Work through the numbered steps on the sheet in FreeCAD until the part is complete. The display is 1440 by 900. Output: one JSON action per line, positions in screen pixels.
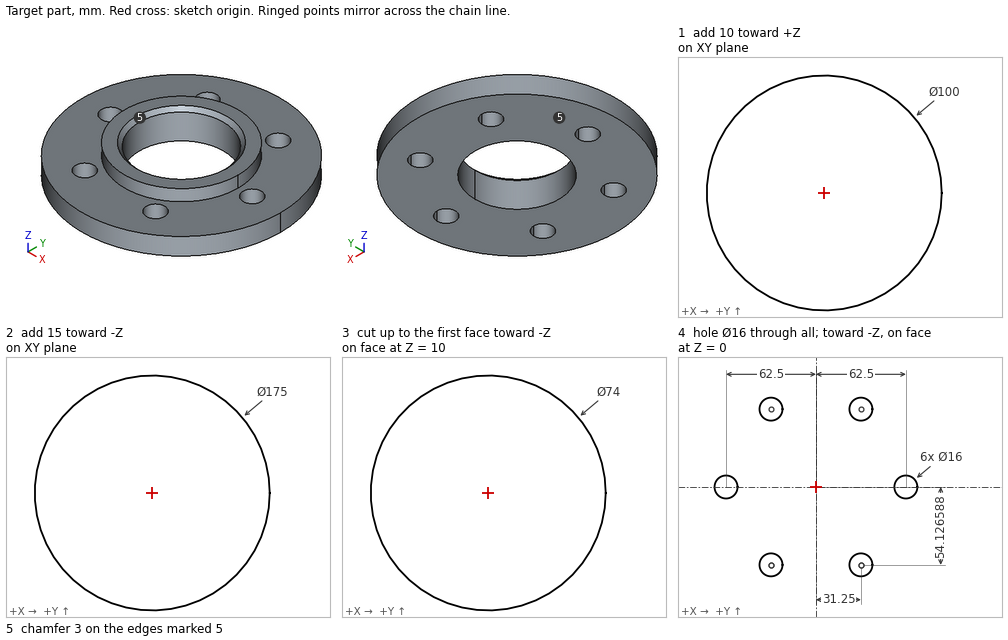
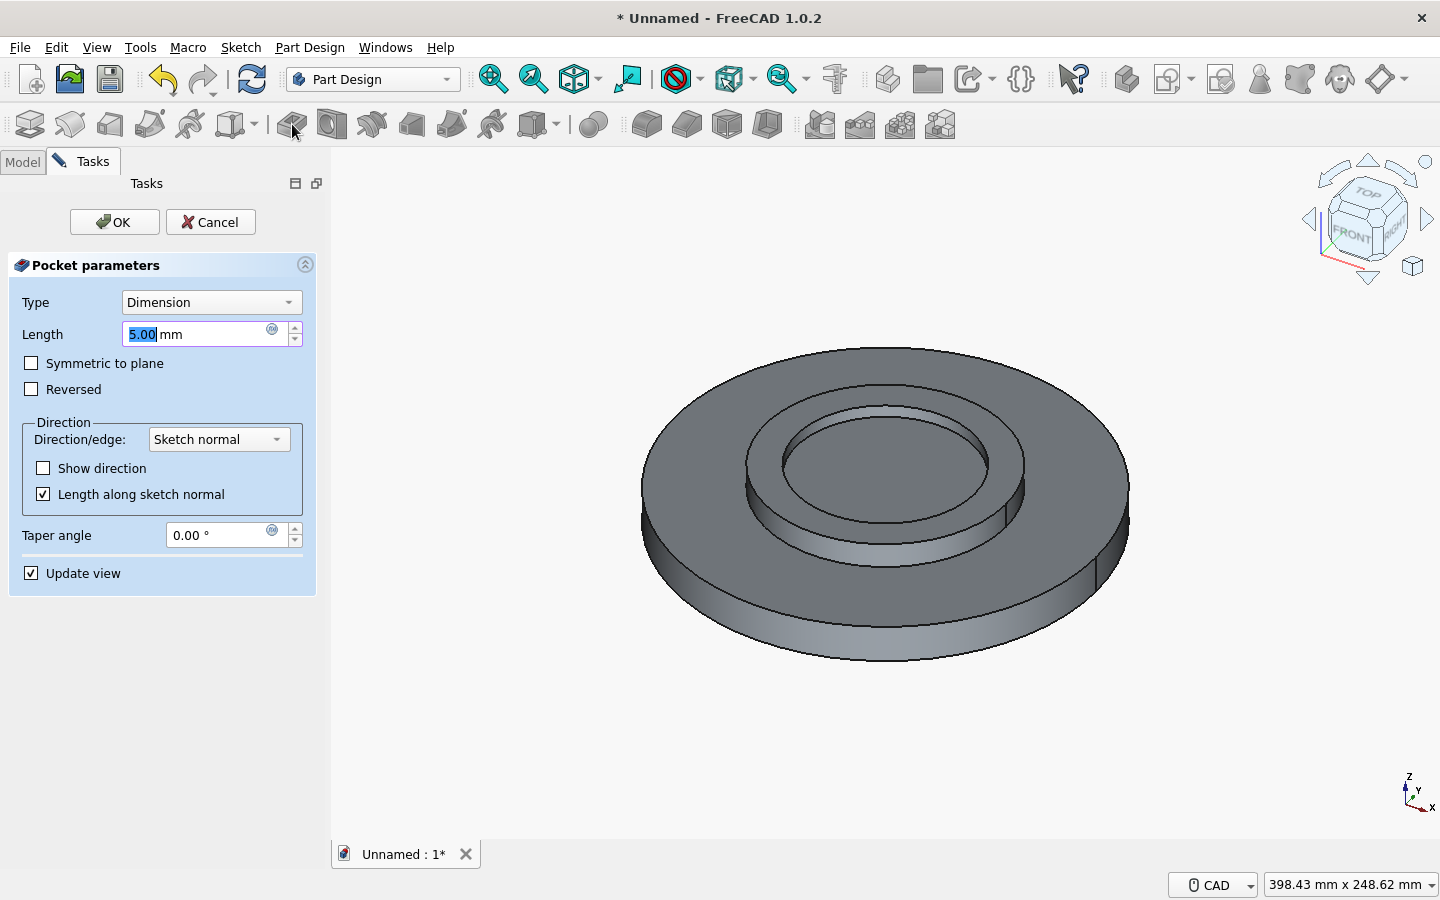
{"action": "left_click", "coordinate": [212, 302]}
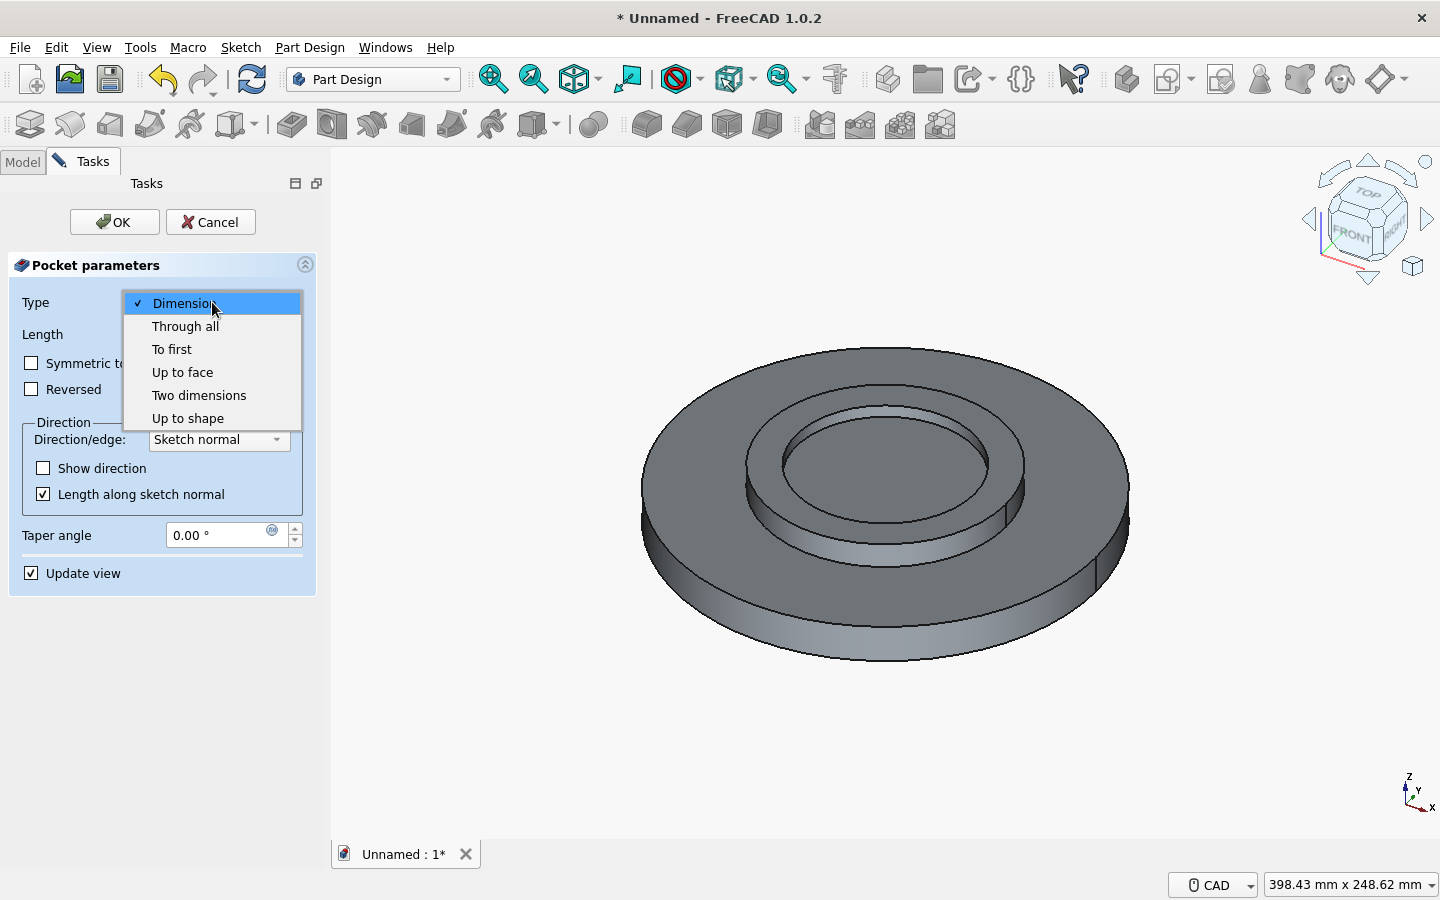
{"action": "left_click", "coordinate": [212, 350]}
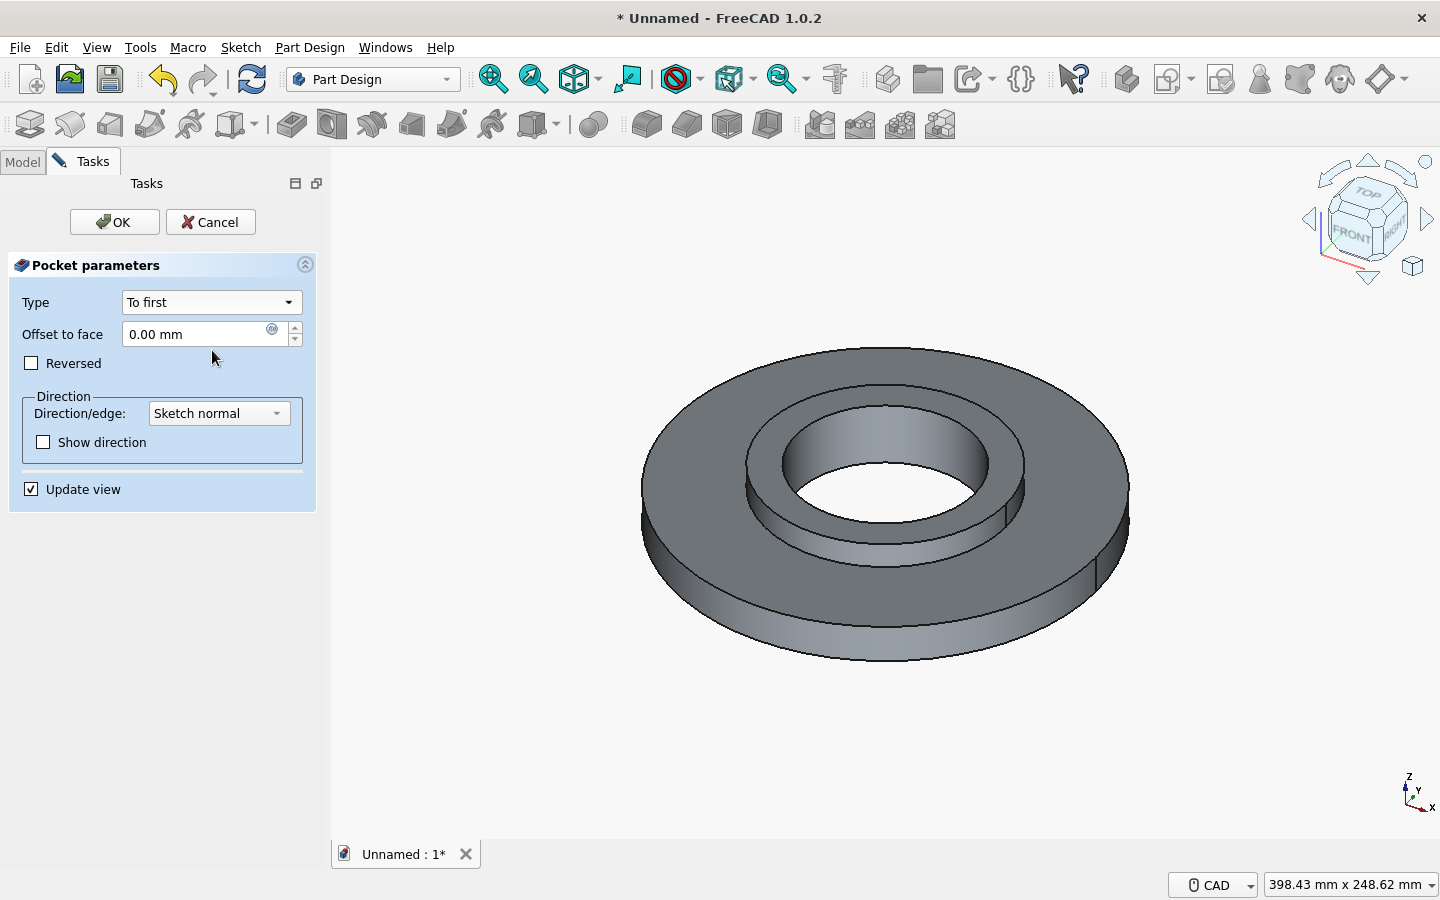
{"action": "left_click", "coordinate": [115, 222]}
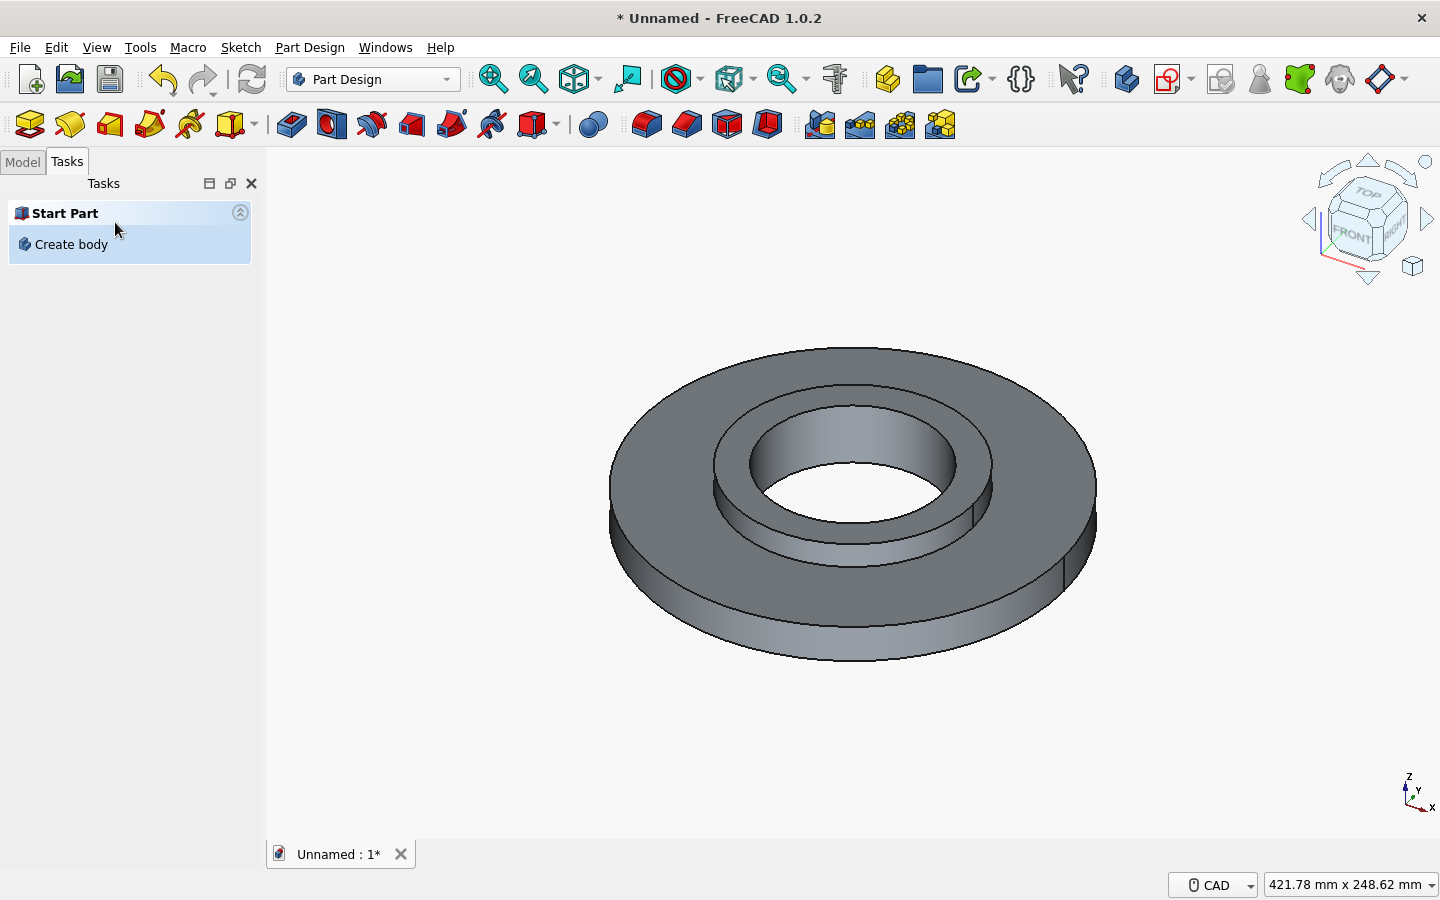
{"action": "left_click", "coordinate": [904, 595]}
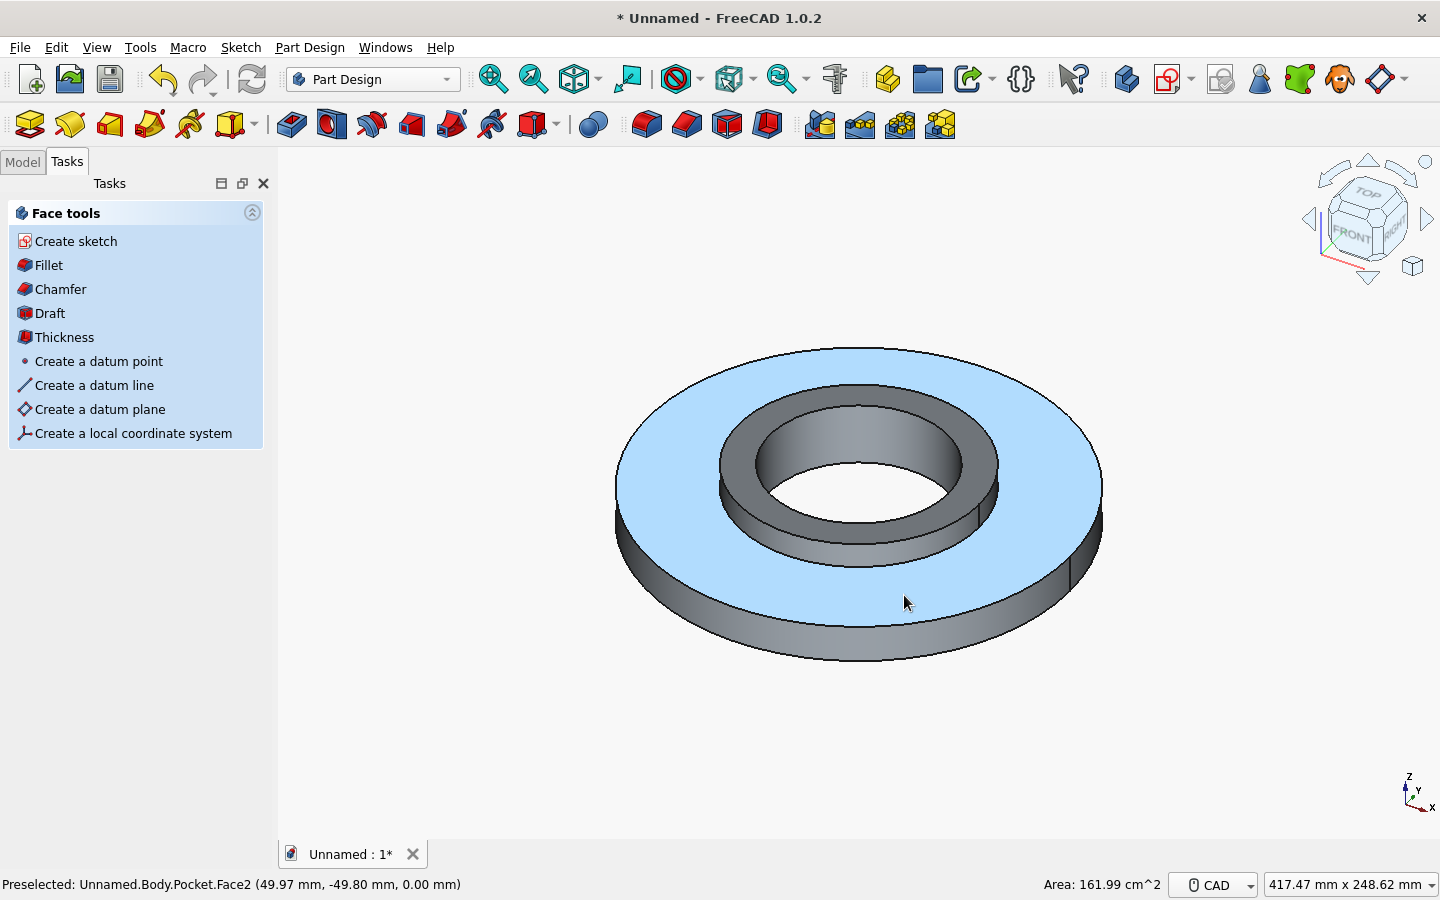
{"action": "left_click", "coordinate": [1168, 80]}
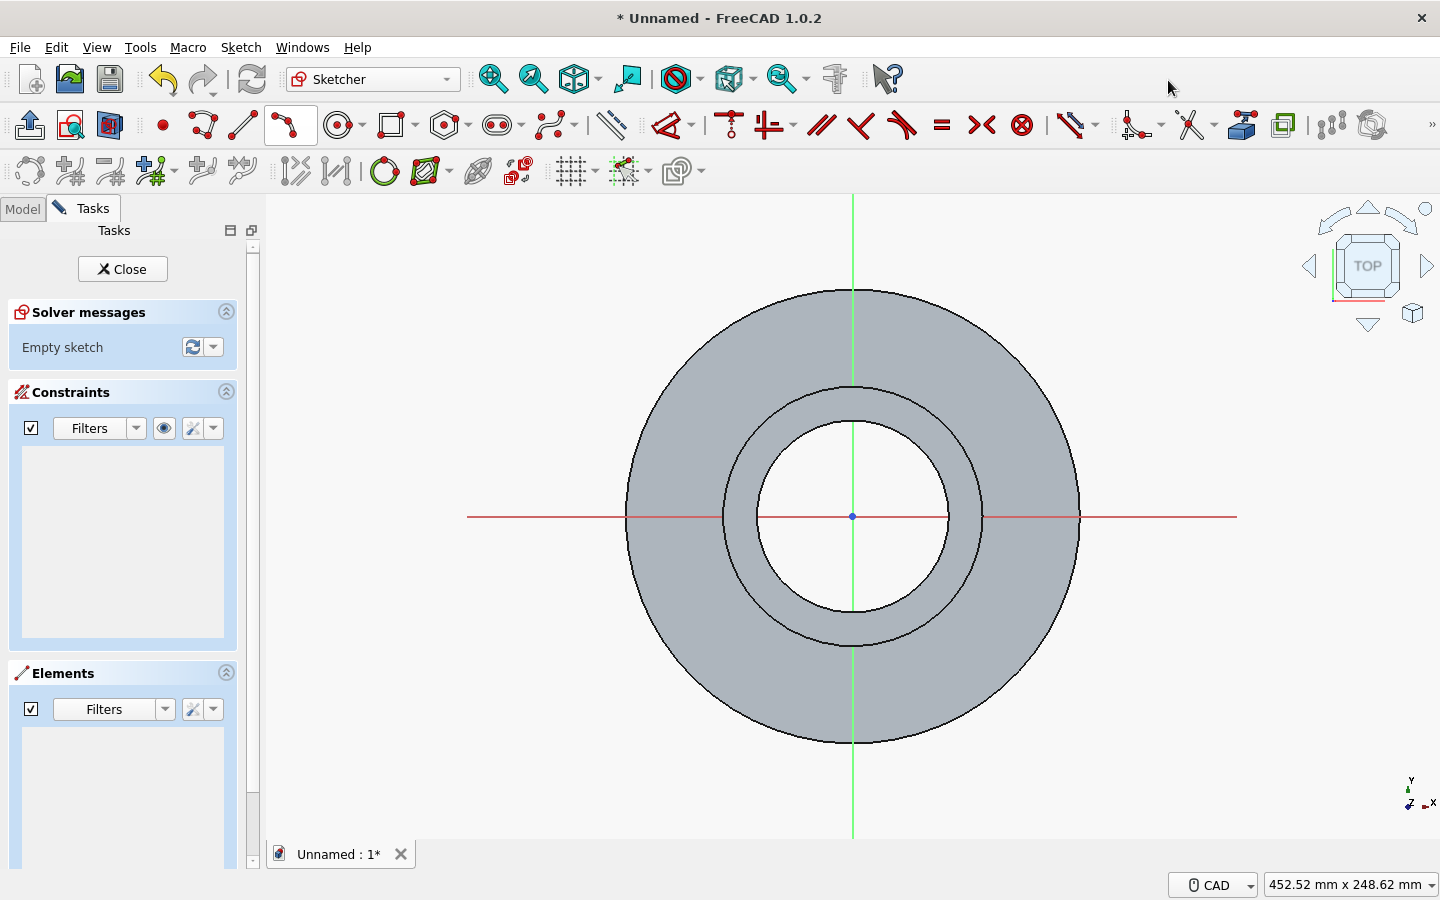
{"action": "left_click", "coordinate": [338, 126]}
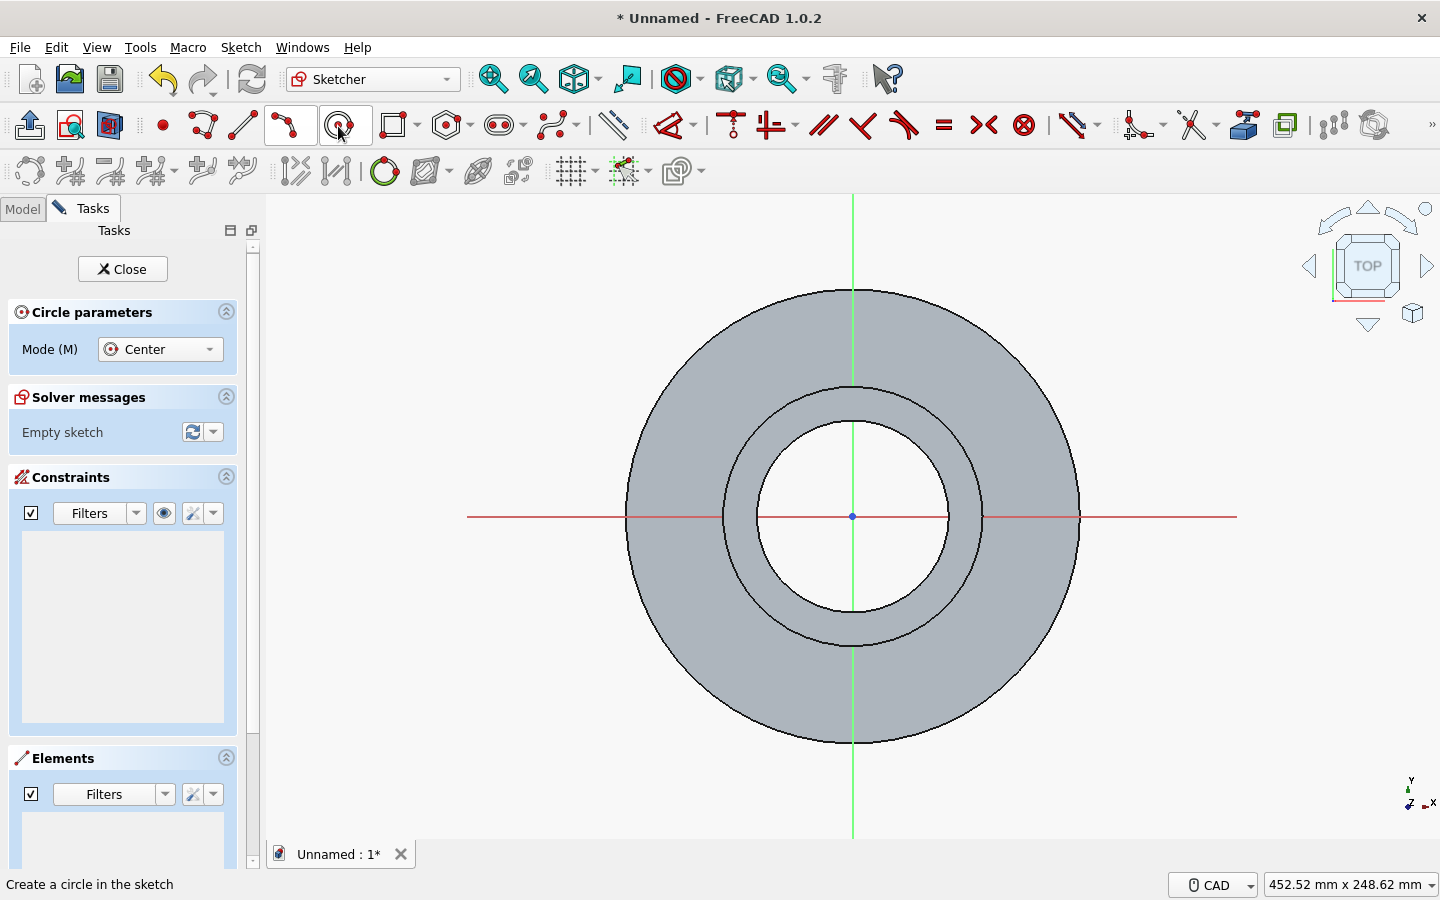
{"action": "left_click", "coordinate": [1015, 516]}
{"action": "left_click", "coordinate": [1030, 502]}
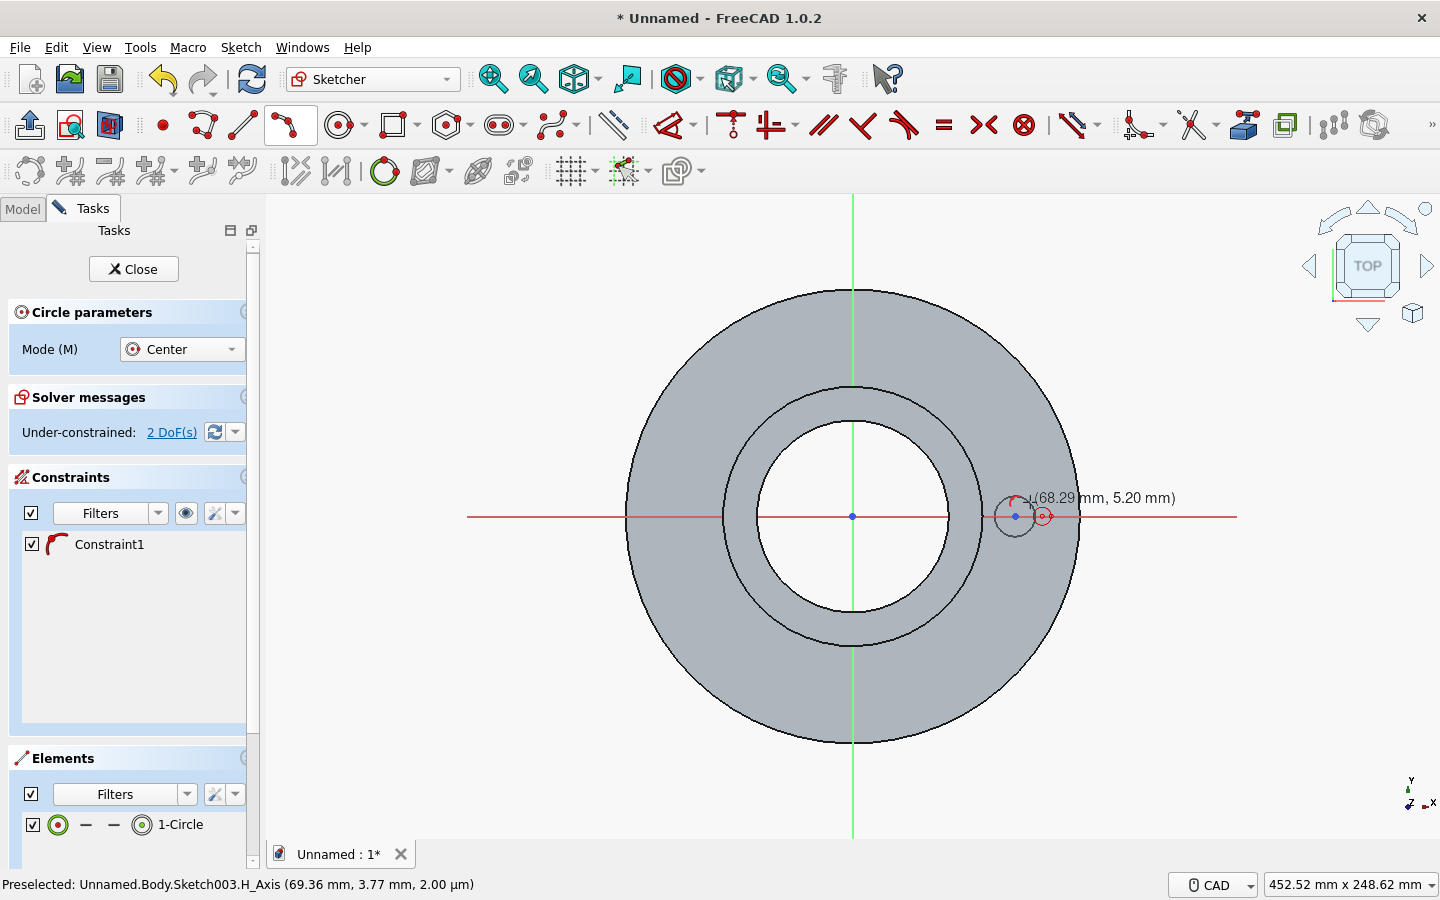
{"action": "left_click", "coordinate": [934, 657]}
{"action": "left_click", "coordinate": [949, 642]}